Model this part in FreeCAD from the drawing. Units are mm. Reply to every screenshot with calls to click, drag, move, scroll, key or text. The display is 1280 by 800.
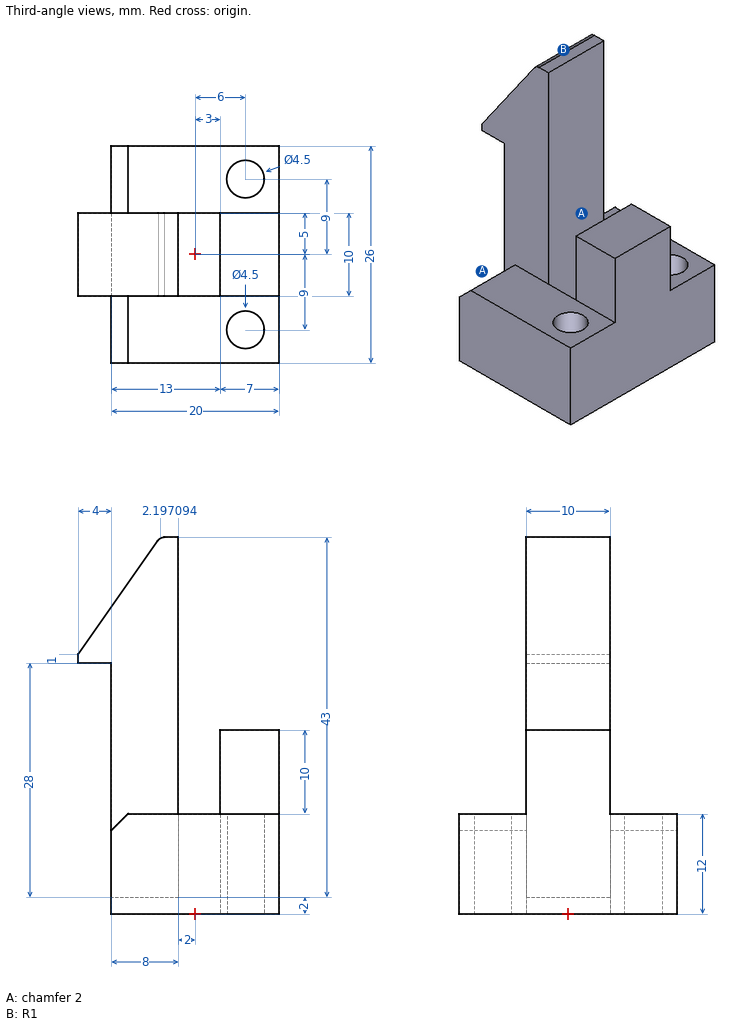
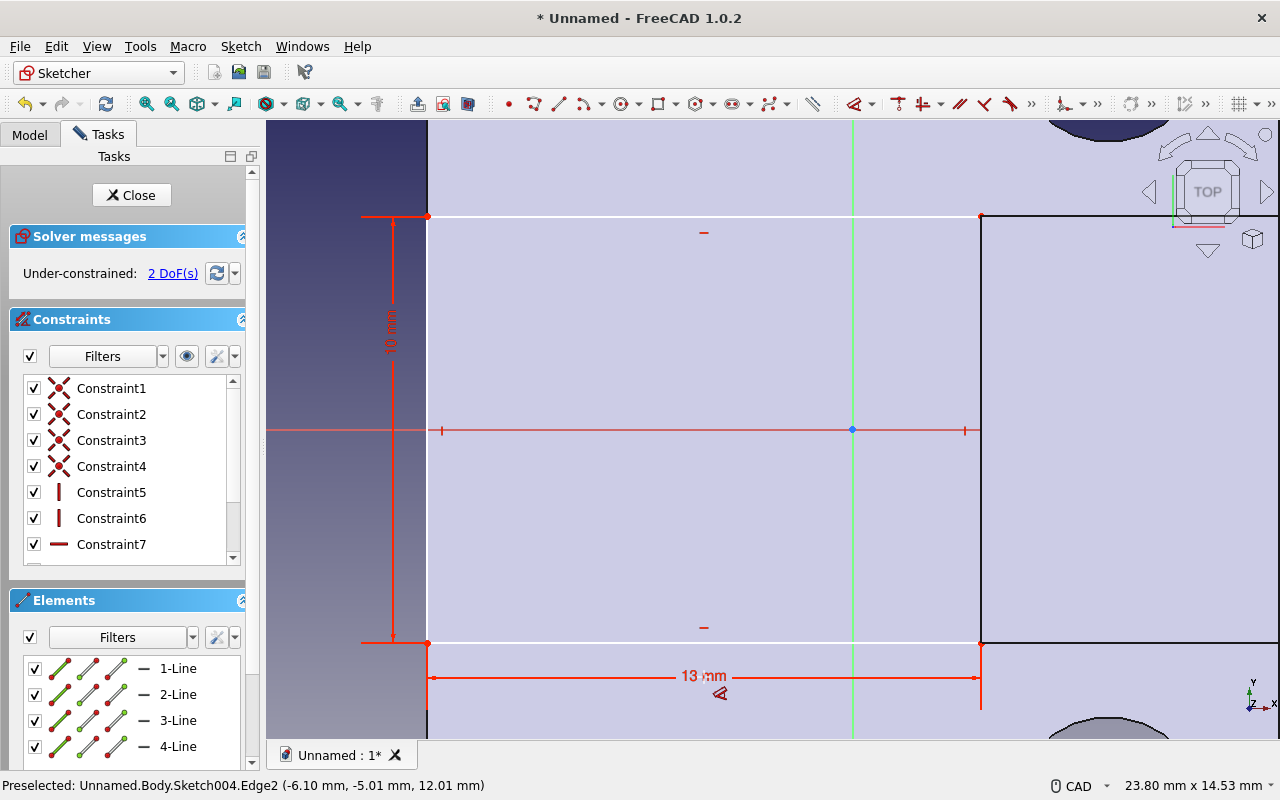
click(427, 217)
click(393, 274)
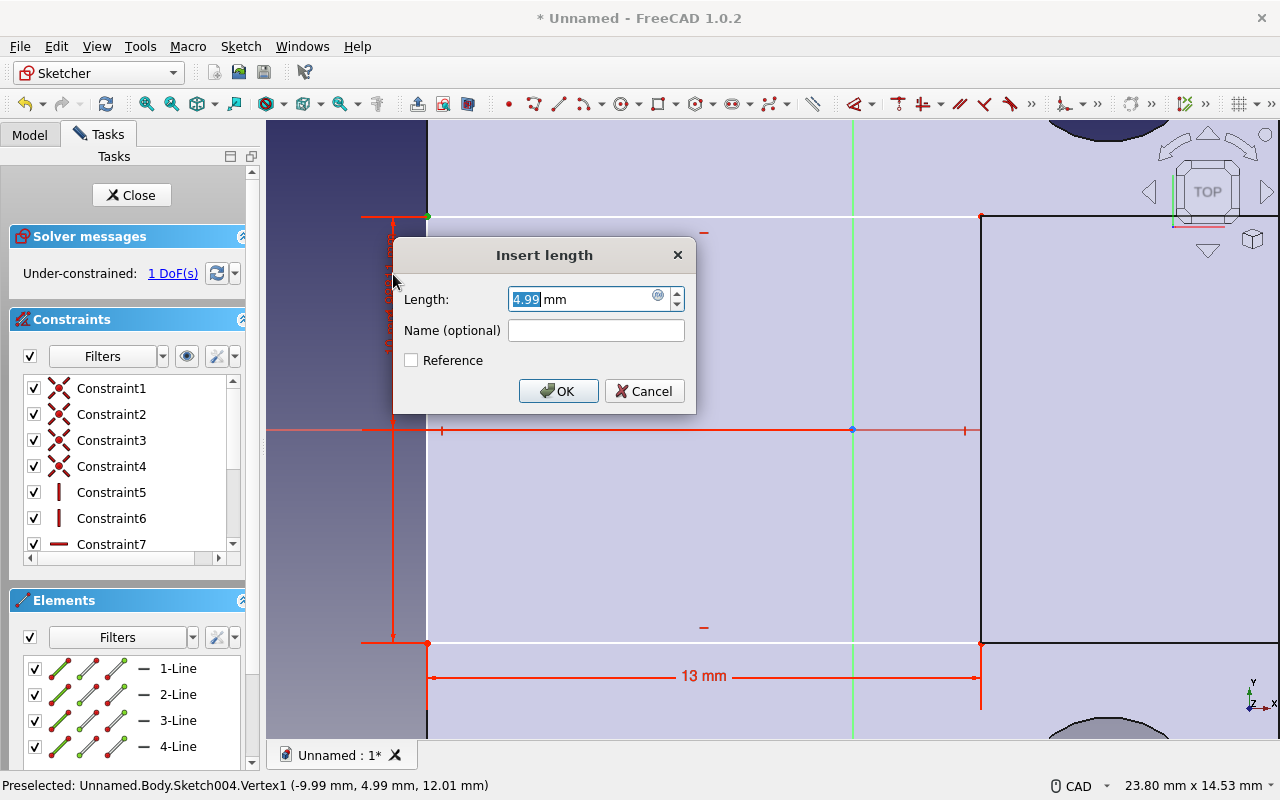
text(5)
key(Return)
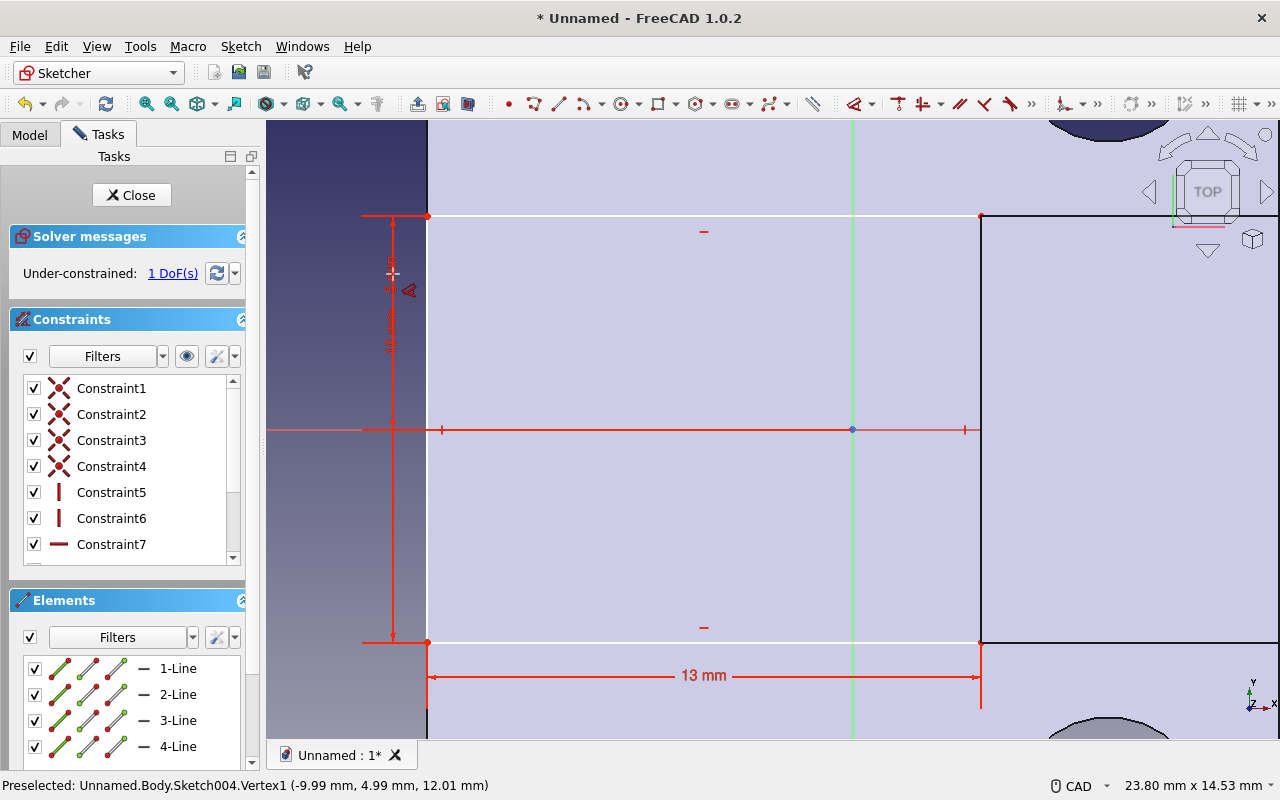
click(981, 643)
click(917, 677)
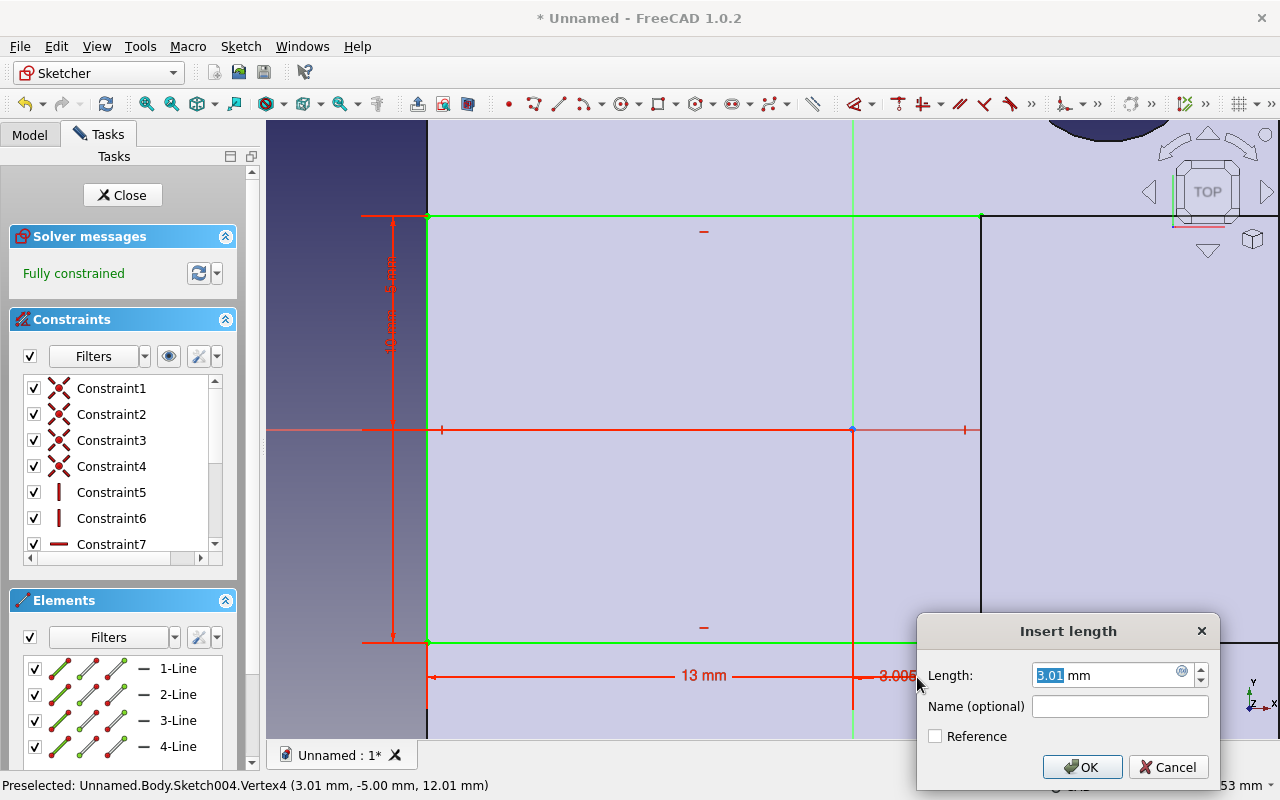
text(3)
key(Return)
key(Escape)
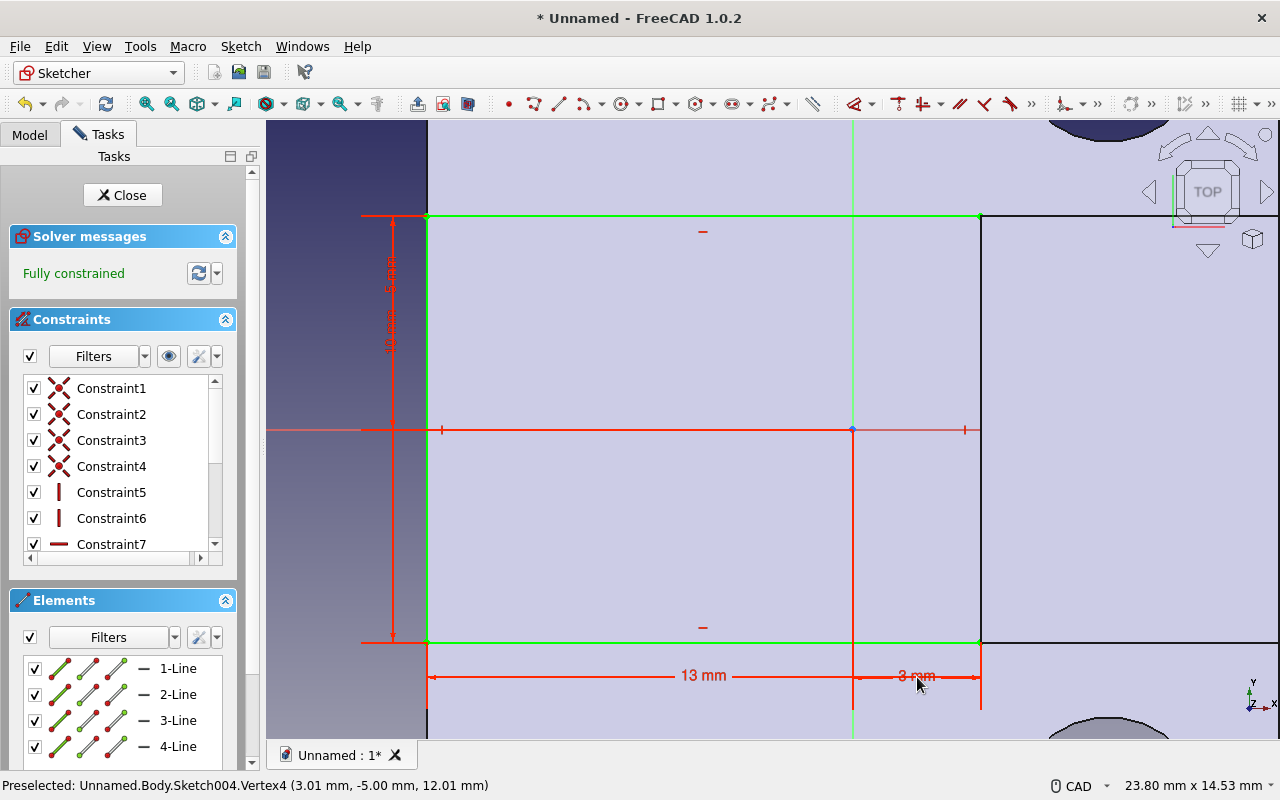
click(123, 195)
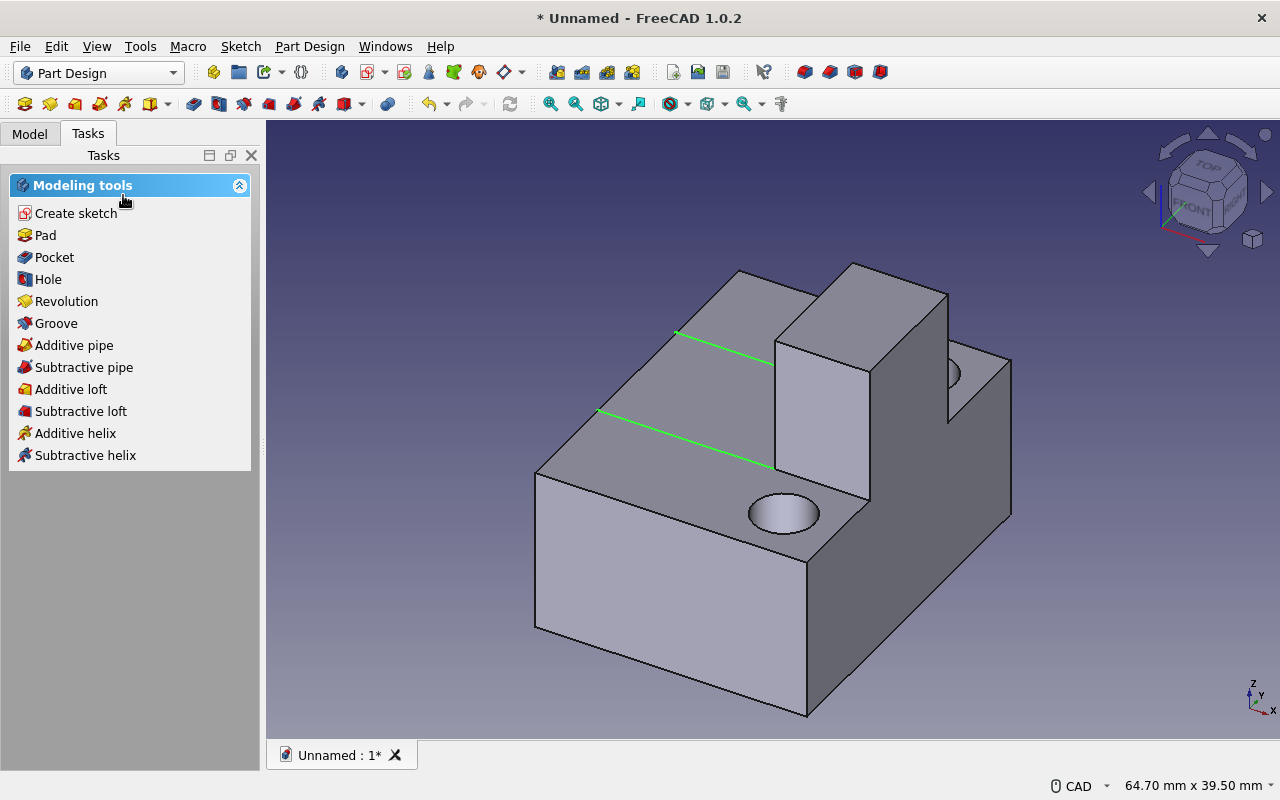
click(194, 104)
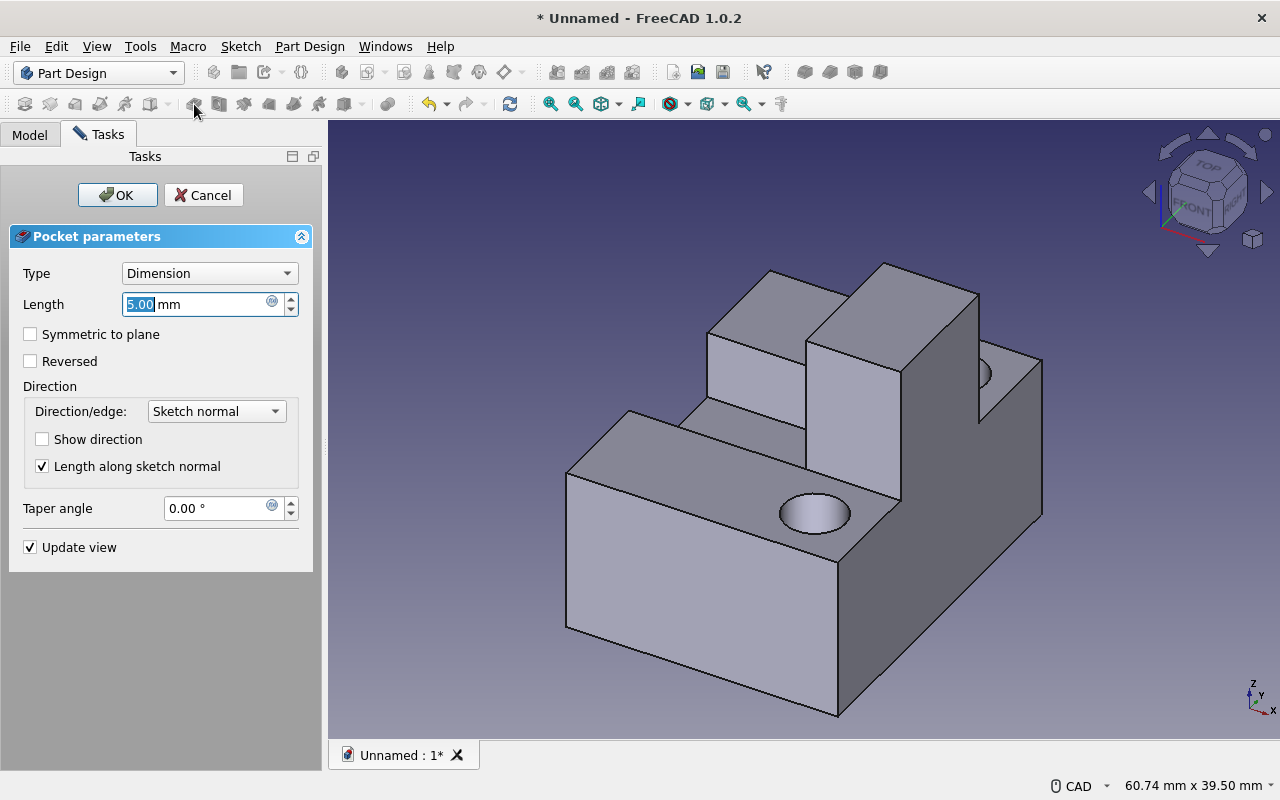
click(210, 274)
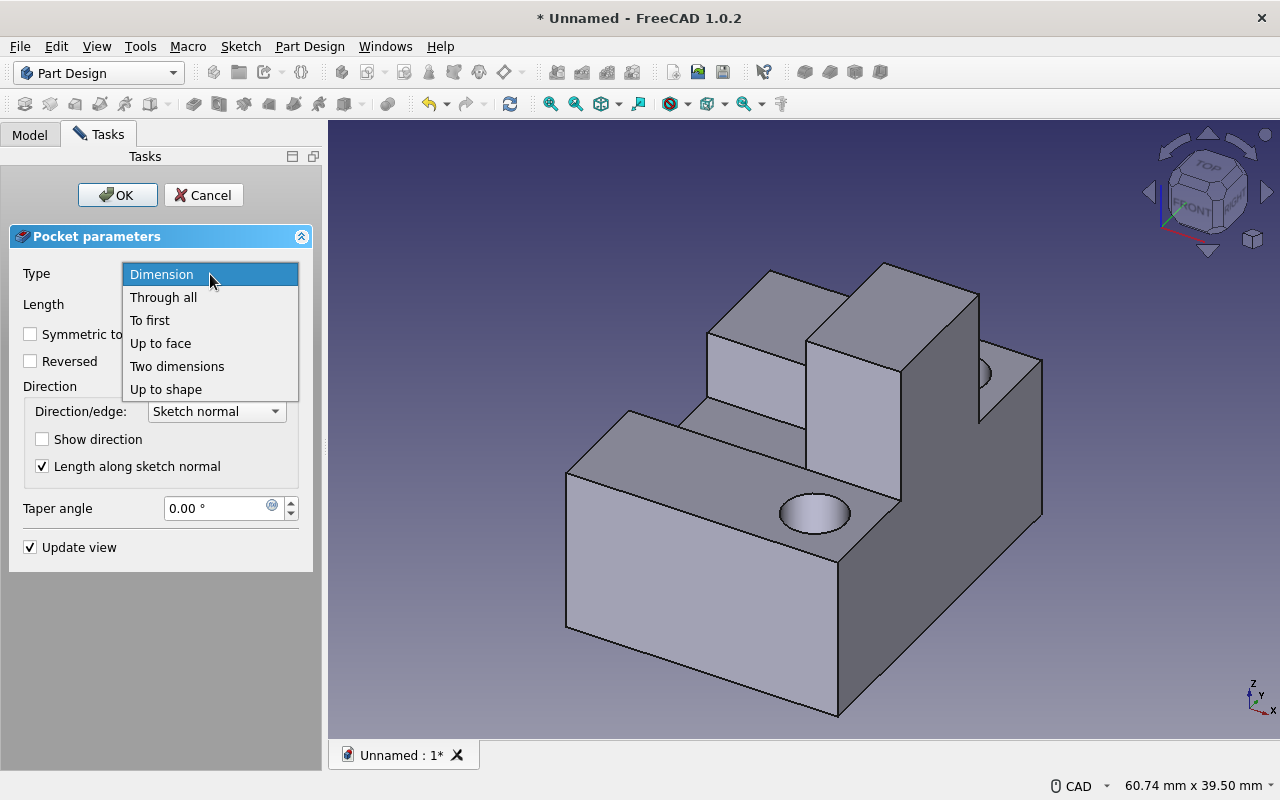
click(208, 320)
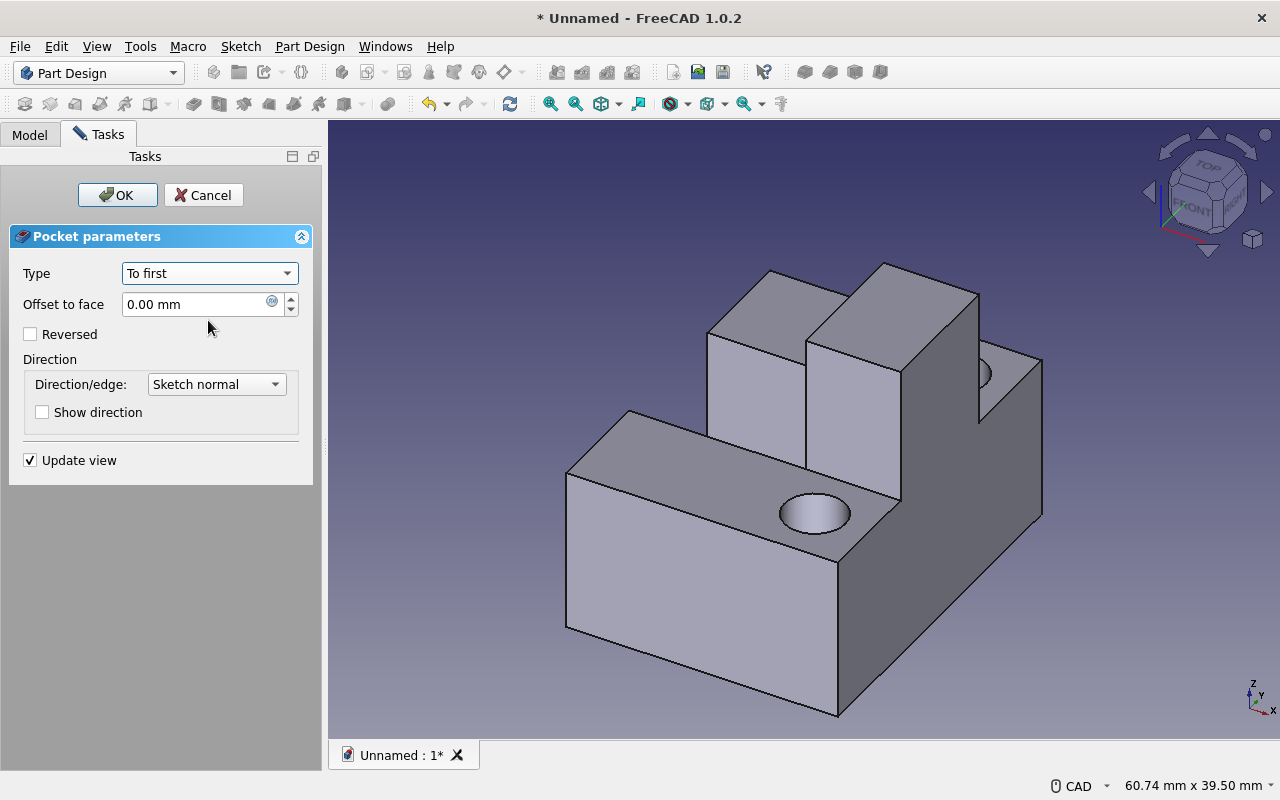
click(118, 195)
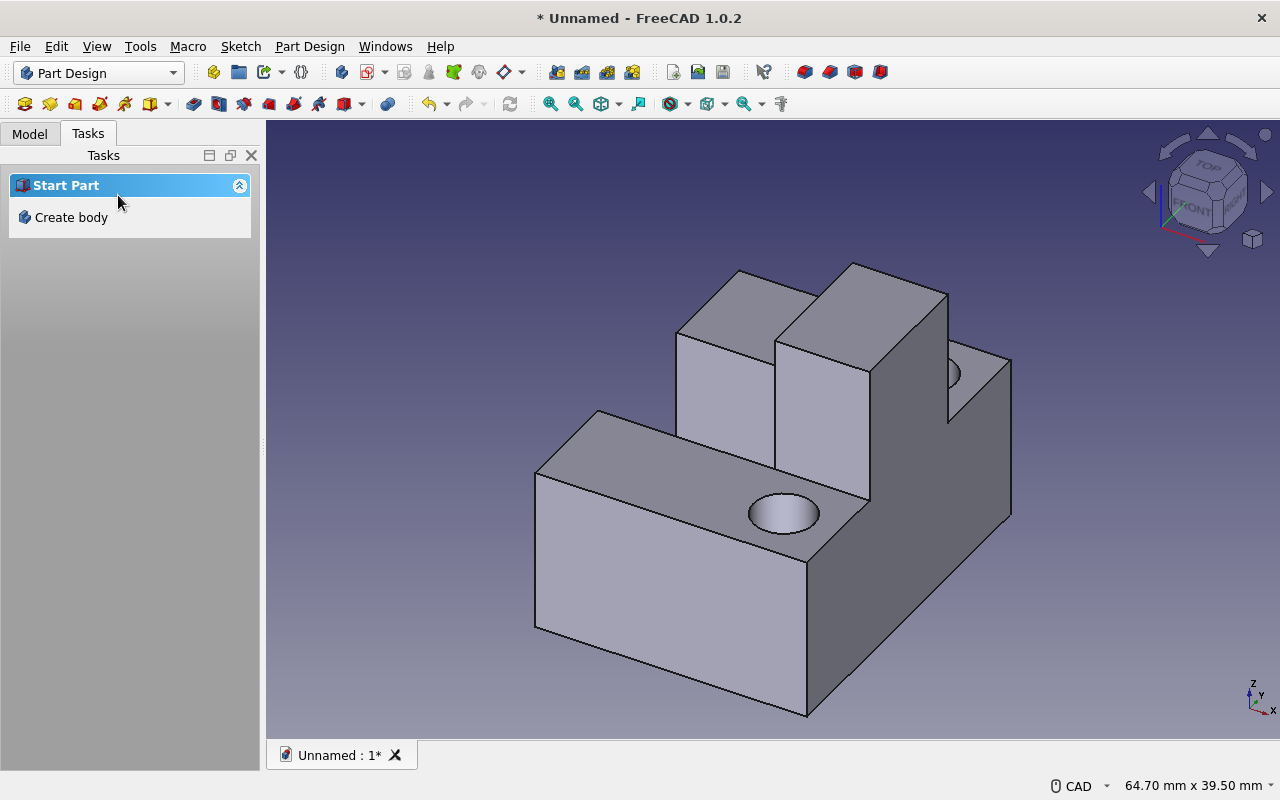
key(0)